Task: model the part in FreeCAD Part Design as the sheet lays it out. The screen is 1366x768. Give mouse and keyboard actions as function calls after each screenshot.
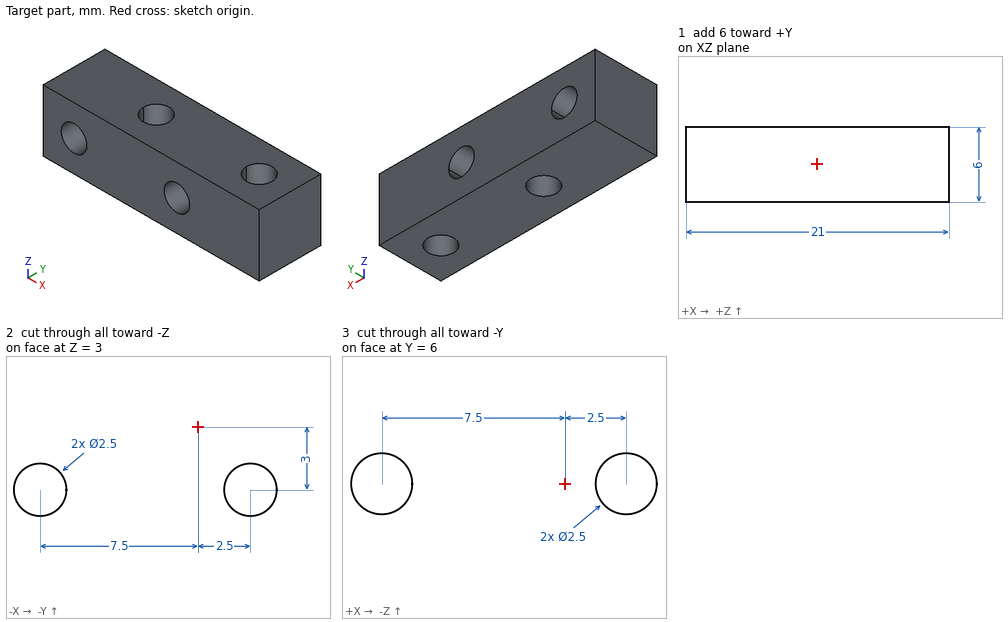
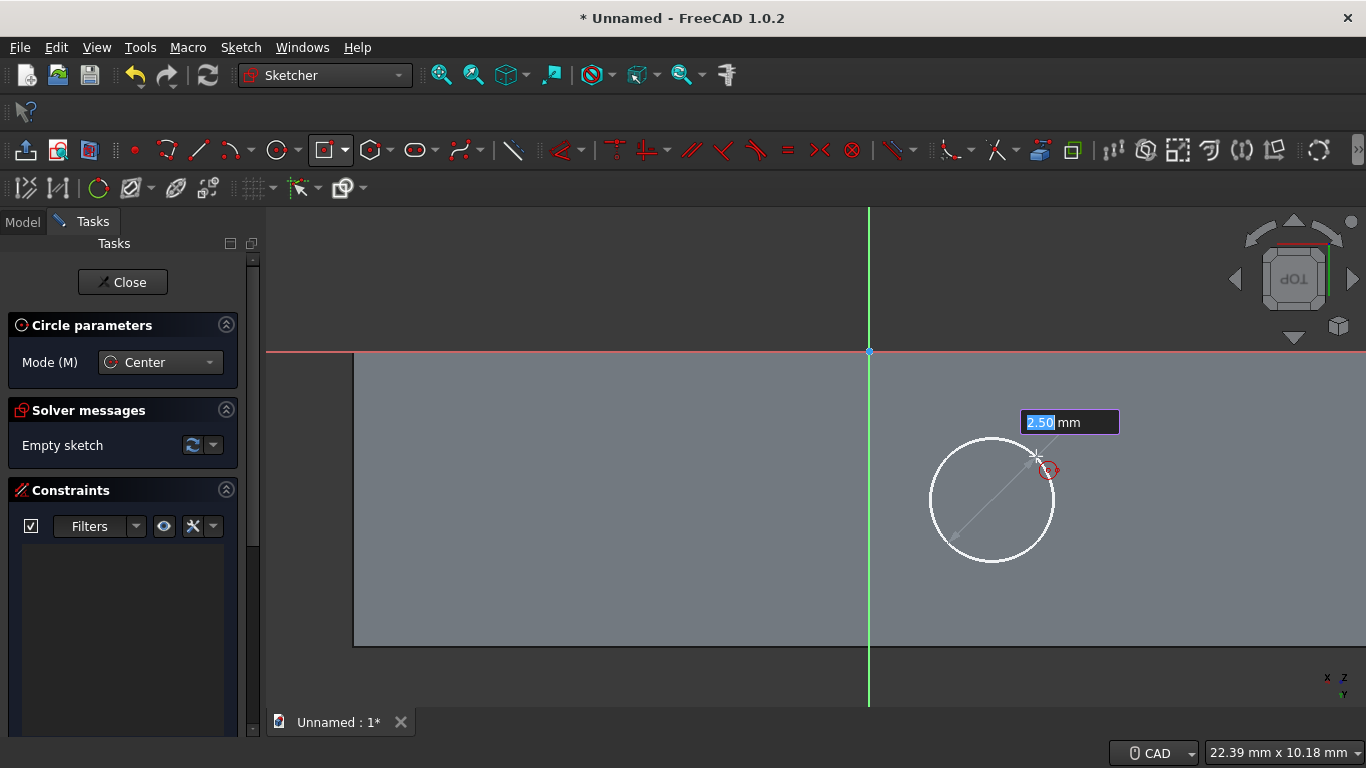
text(2.5)
key(Return)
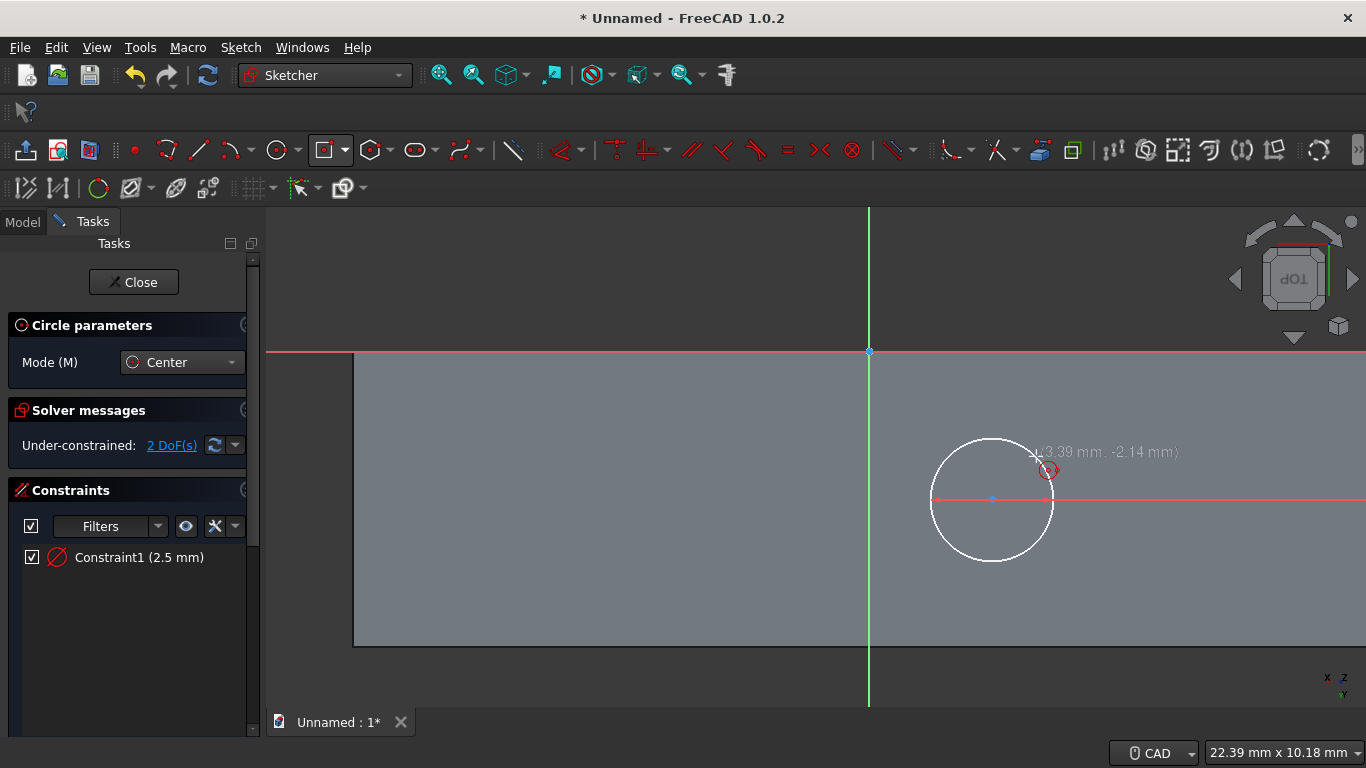
click(501, 499)
move(544, 456)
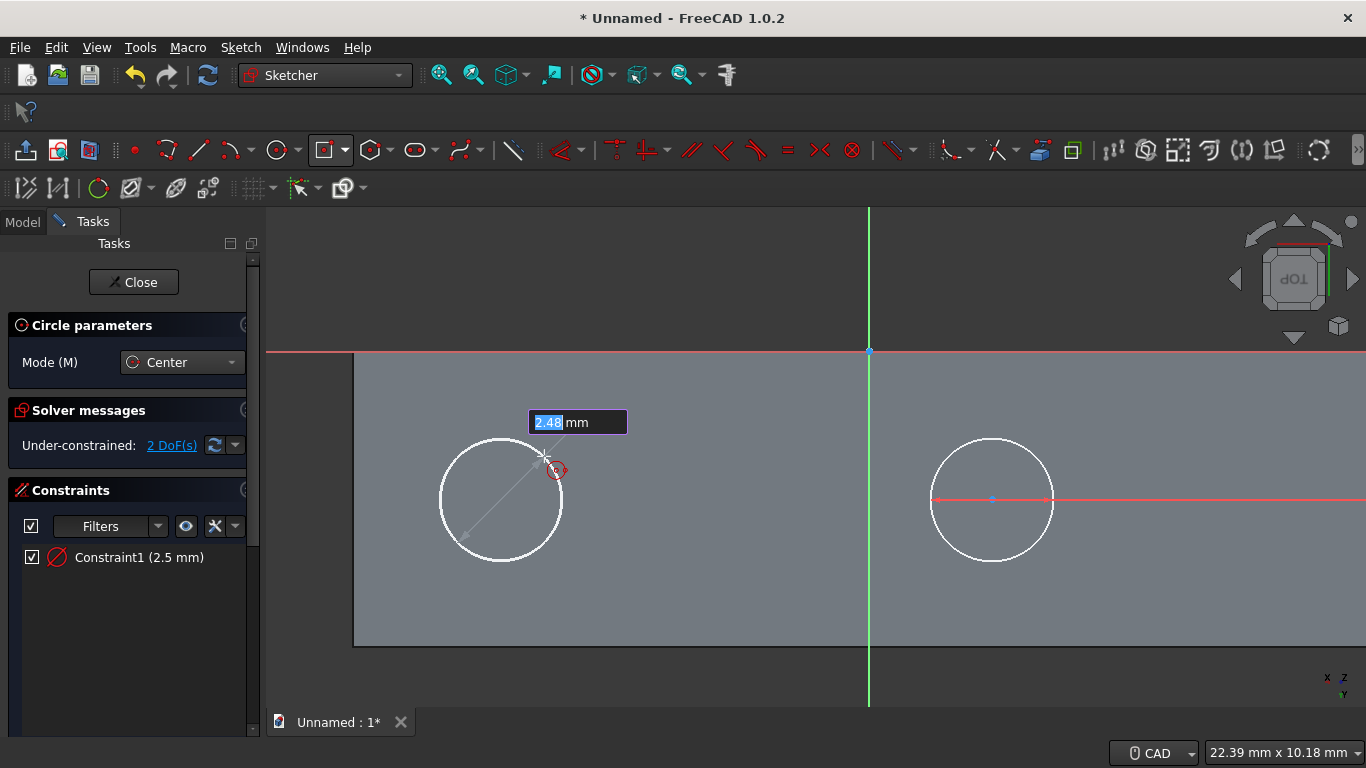
text(2.5)
key(Return)
key(Escape)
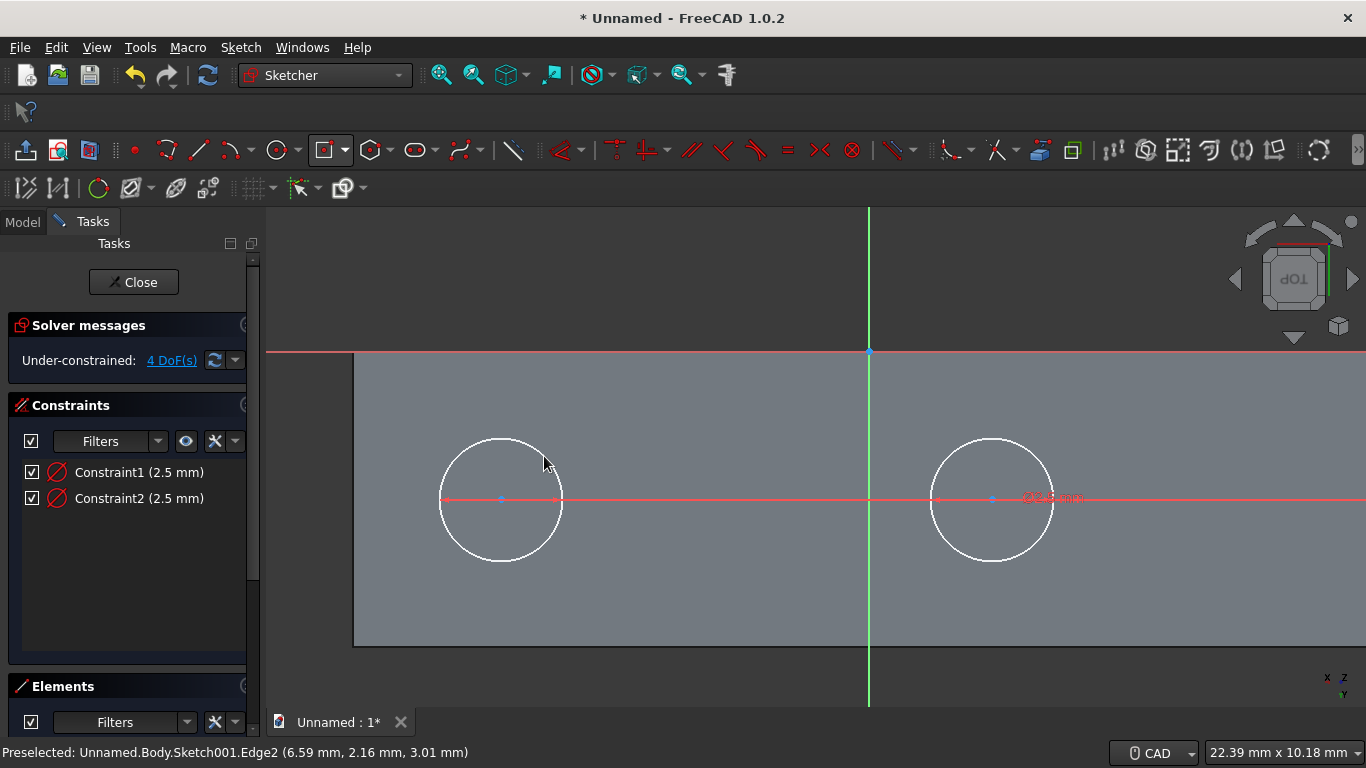
click(992, 500)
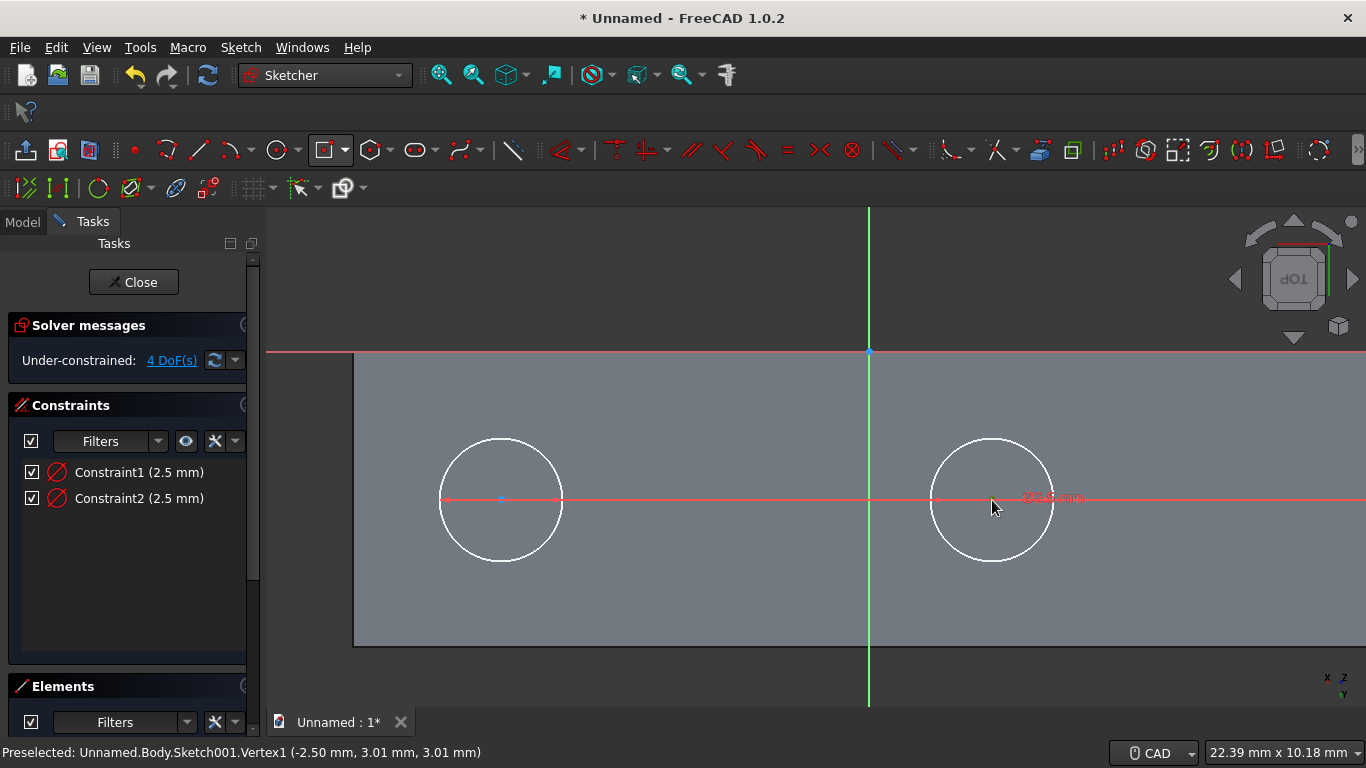
click(501, 500)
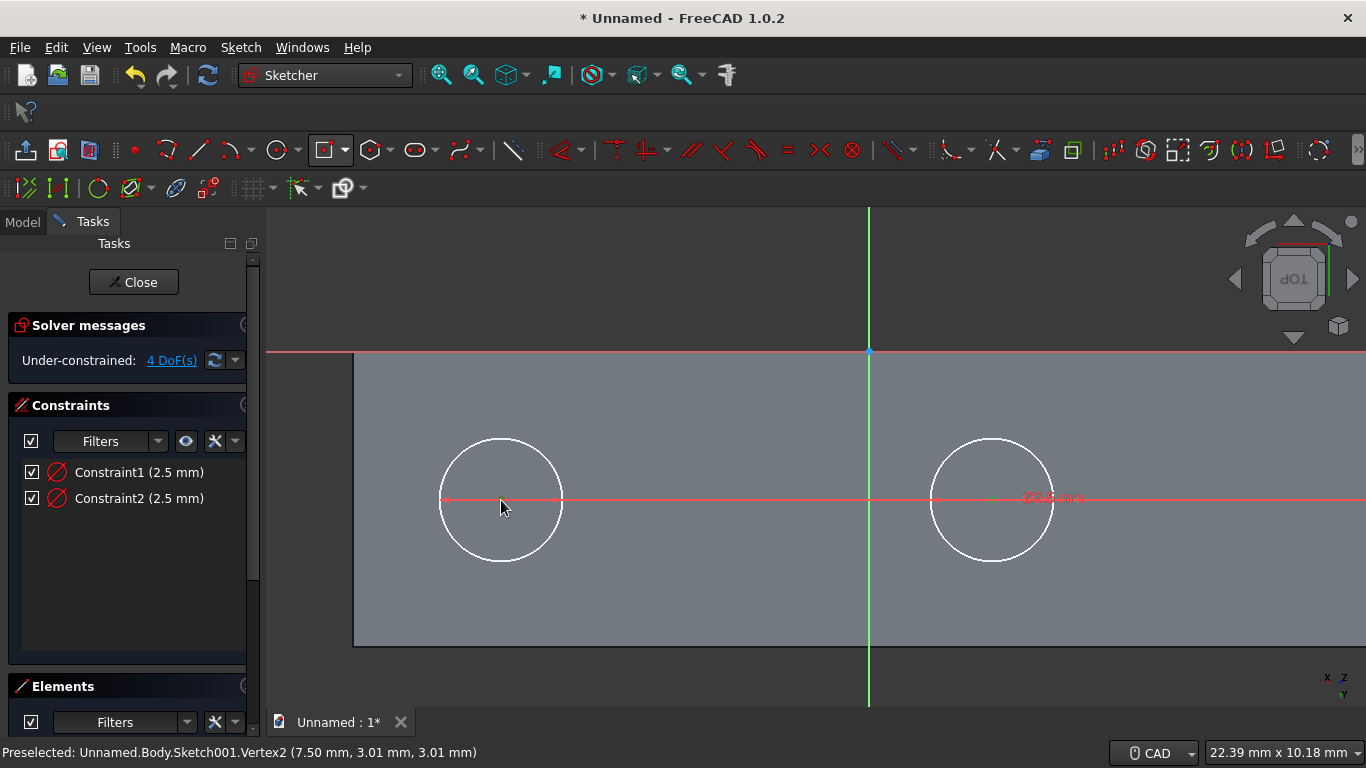
key(h)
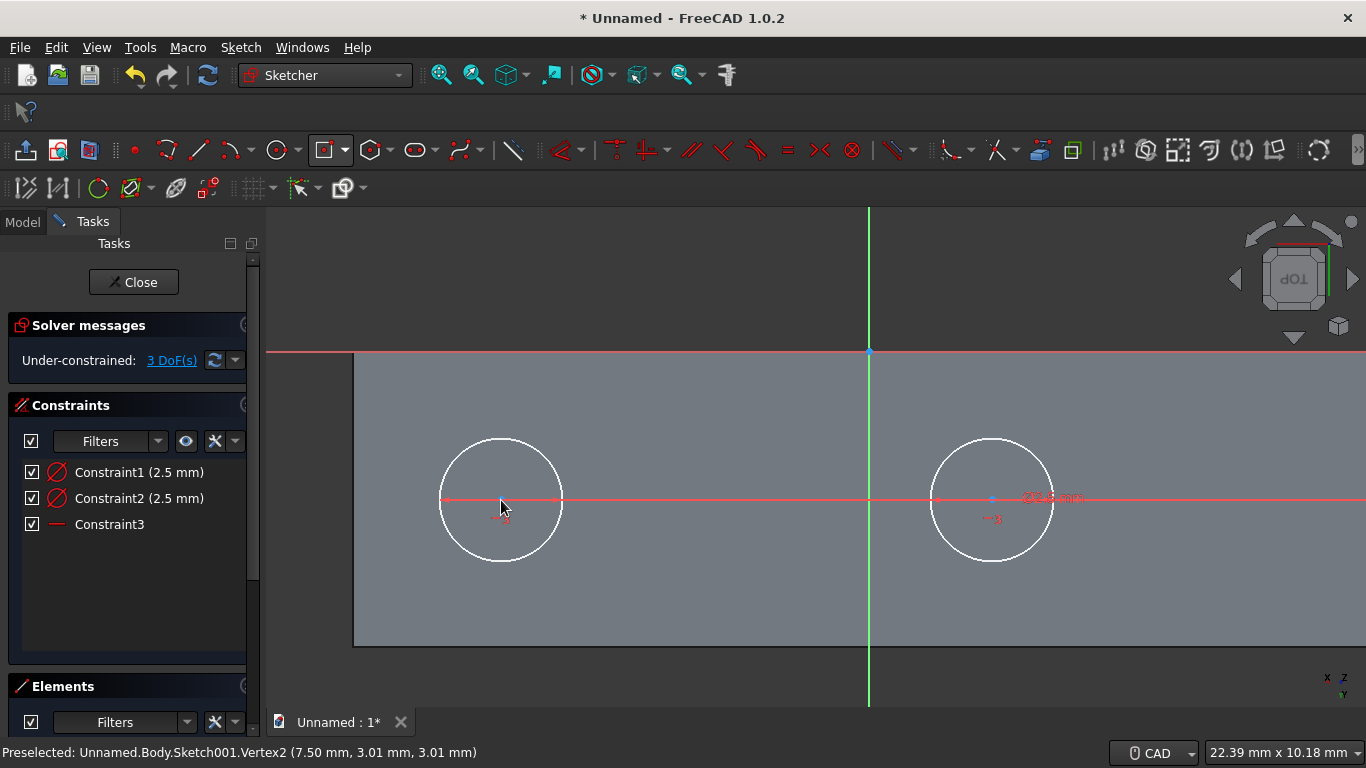
click(560, 150)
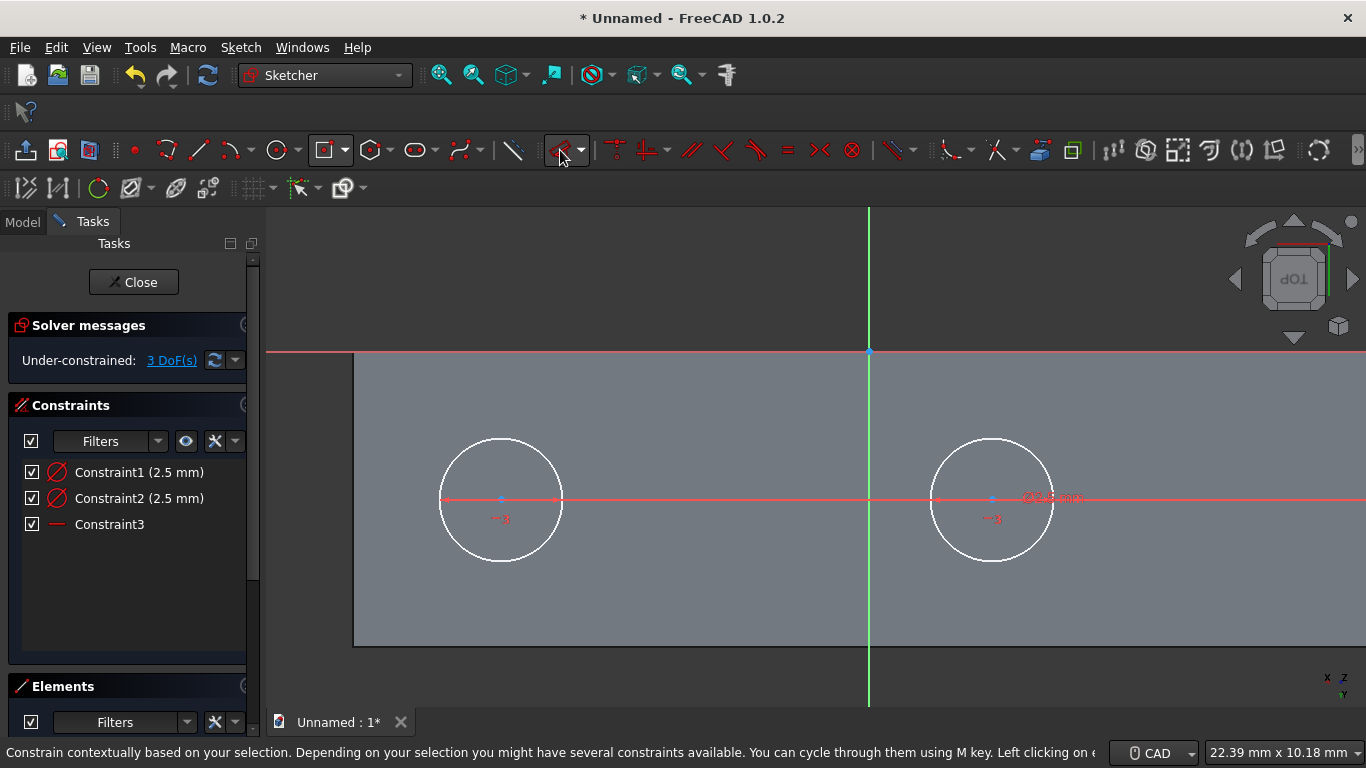
click(992, 500)
click(1026, 426)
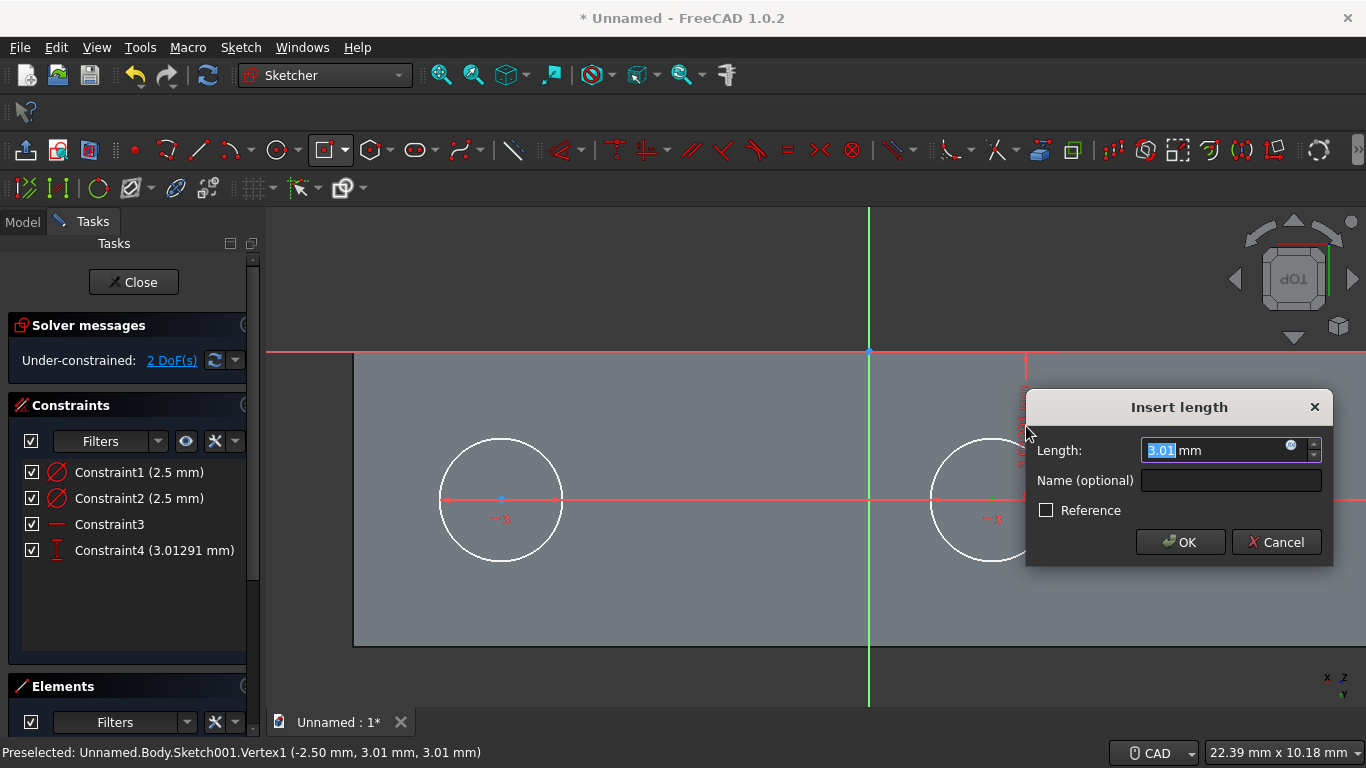
text(3)
key(Return)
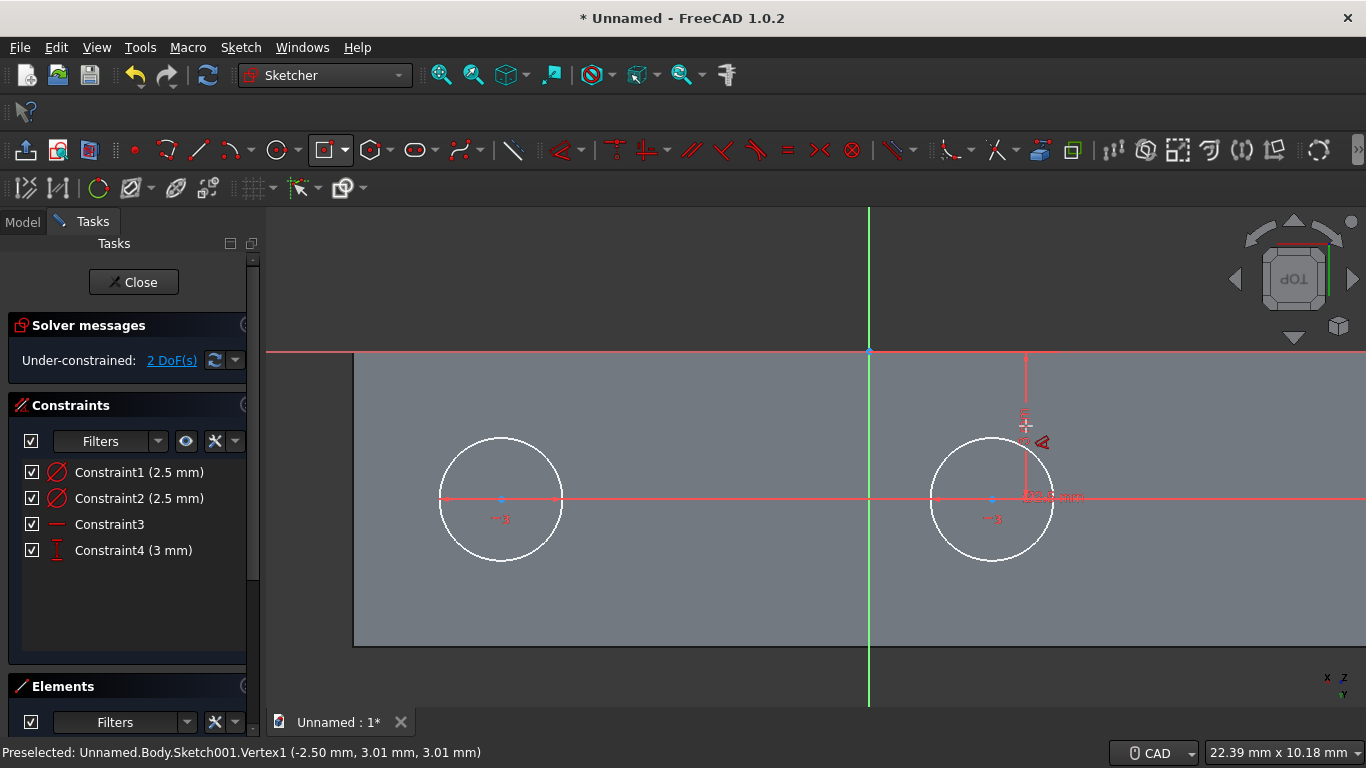
click(992, 499)
click(931, 318)